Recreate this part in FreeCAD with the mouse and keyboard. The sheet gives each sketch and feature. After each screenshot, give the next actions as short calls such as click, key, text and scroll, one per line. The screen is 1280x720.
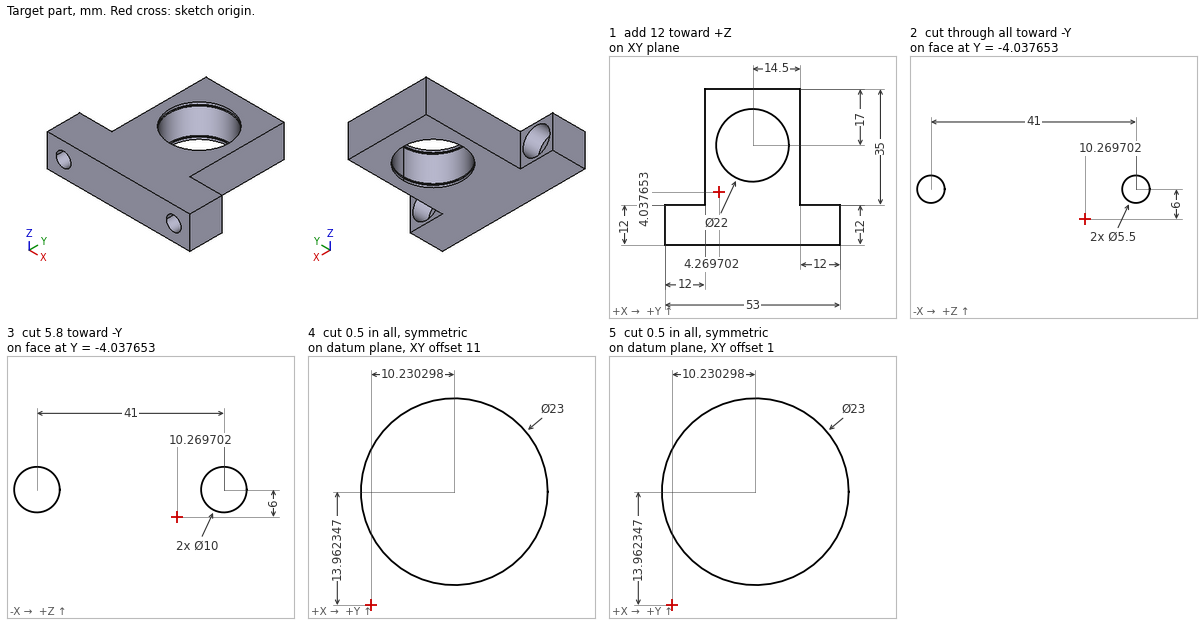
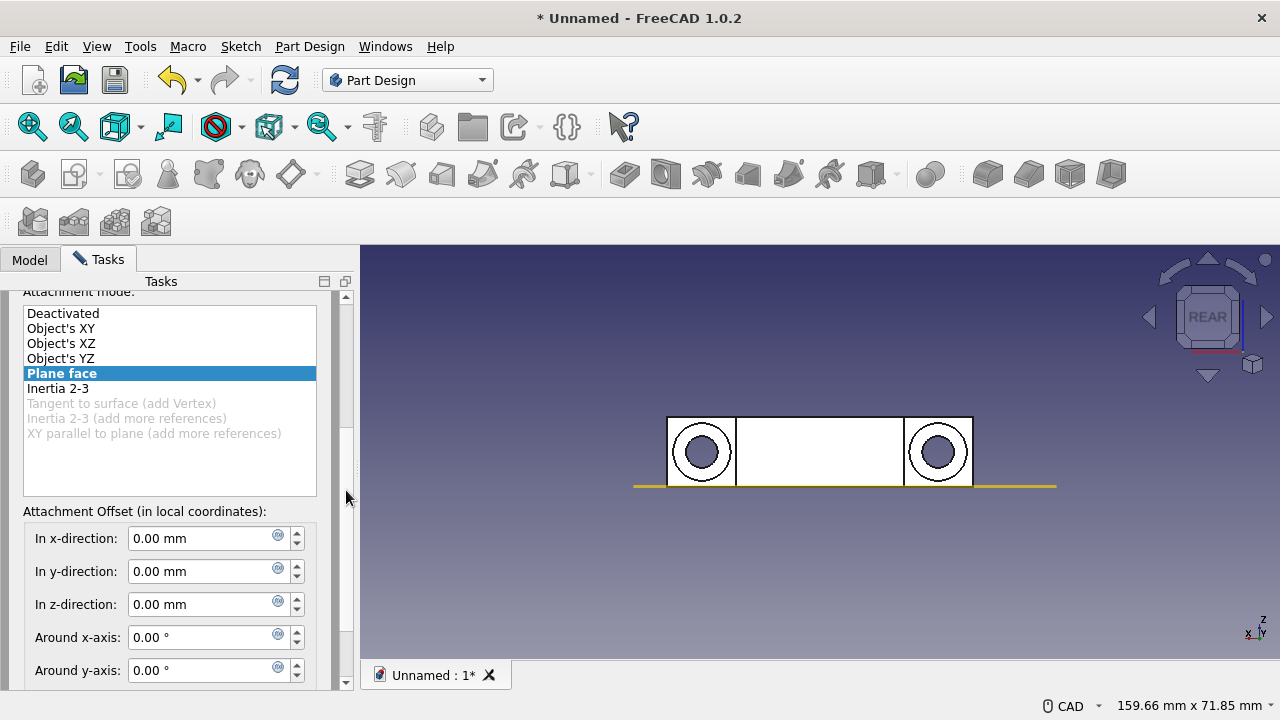
triple_click(210, 604)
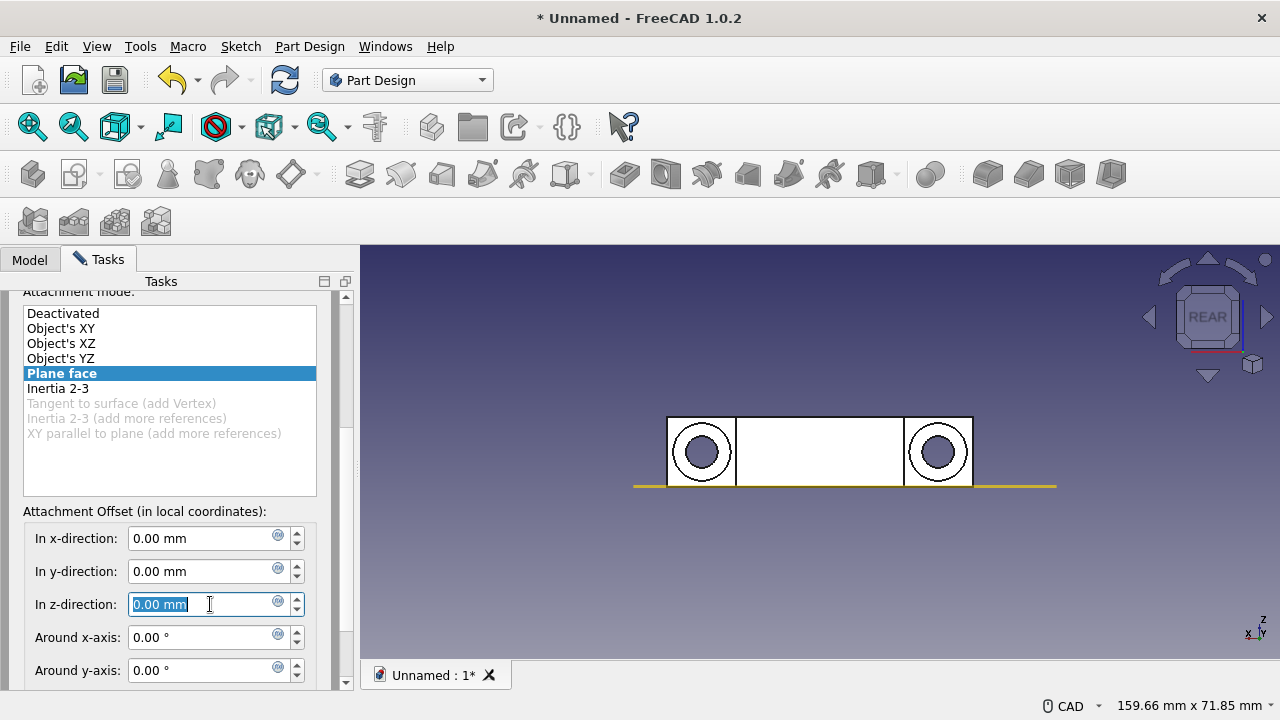
text(1)
key(Tab)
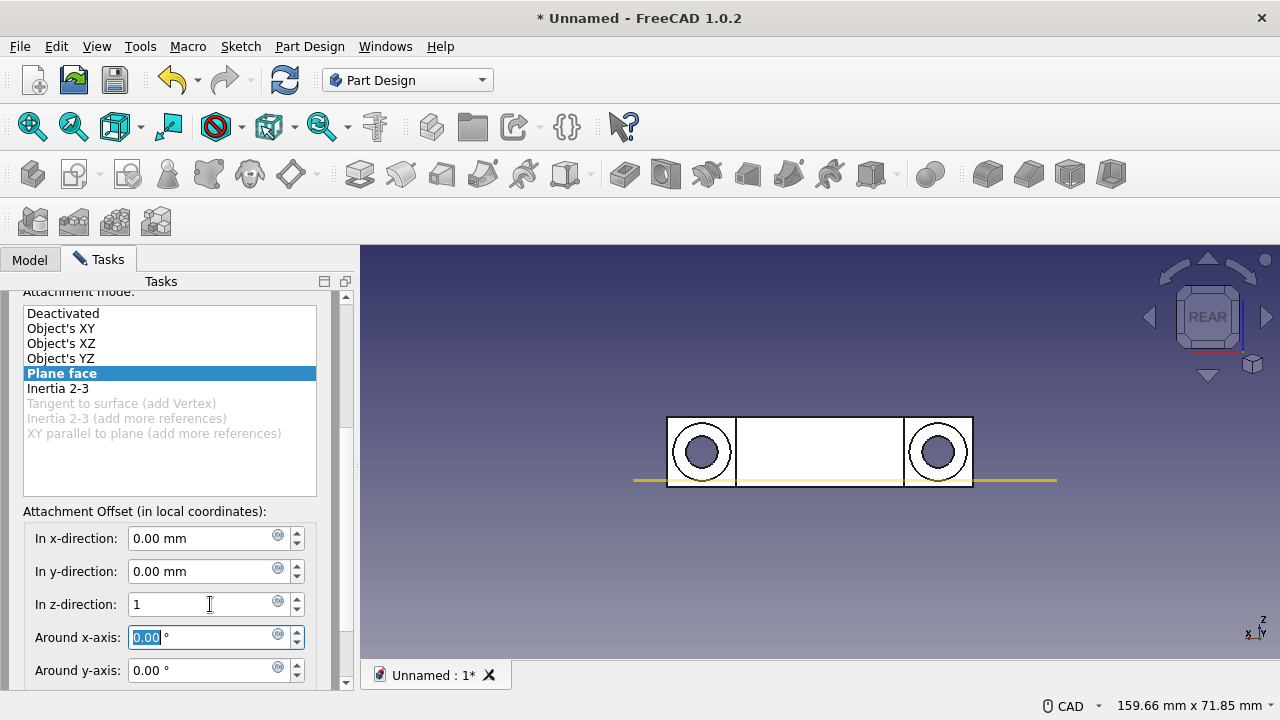
scroll(346, 490, up, 5)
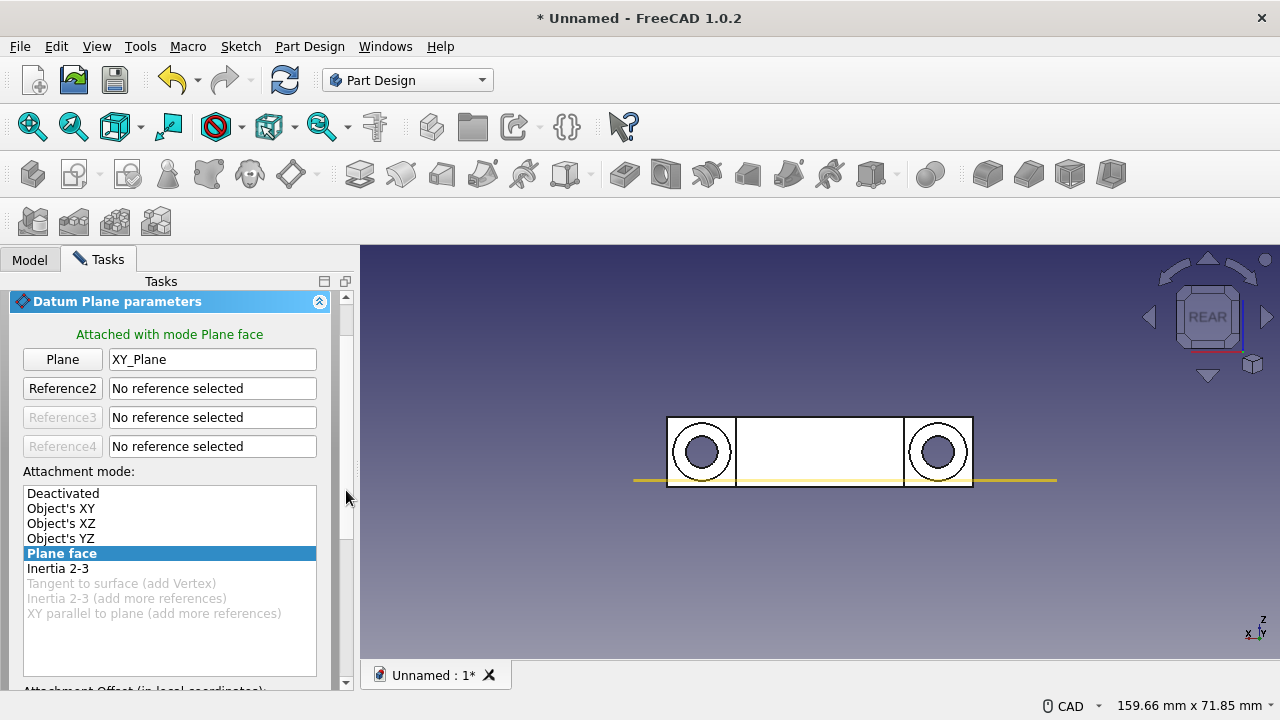
click(127, 320)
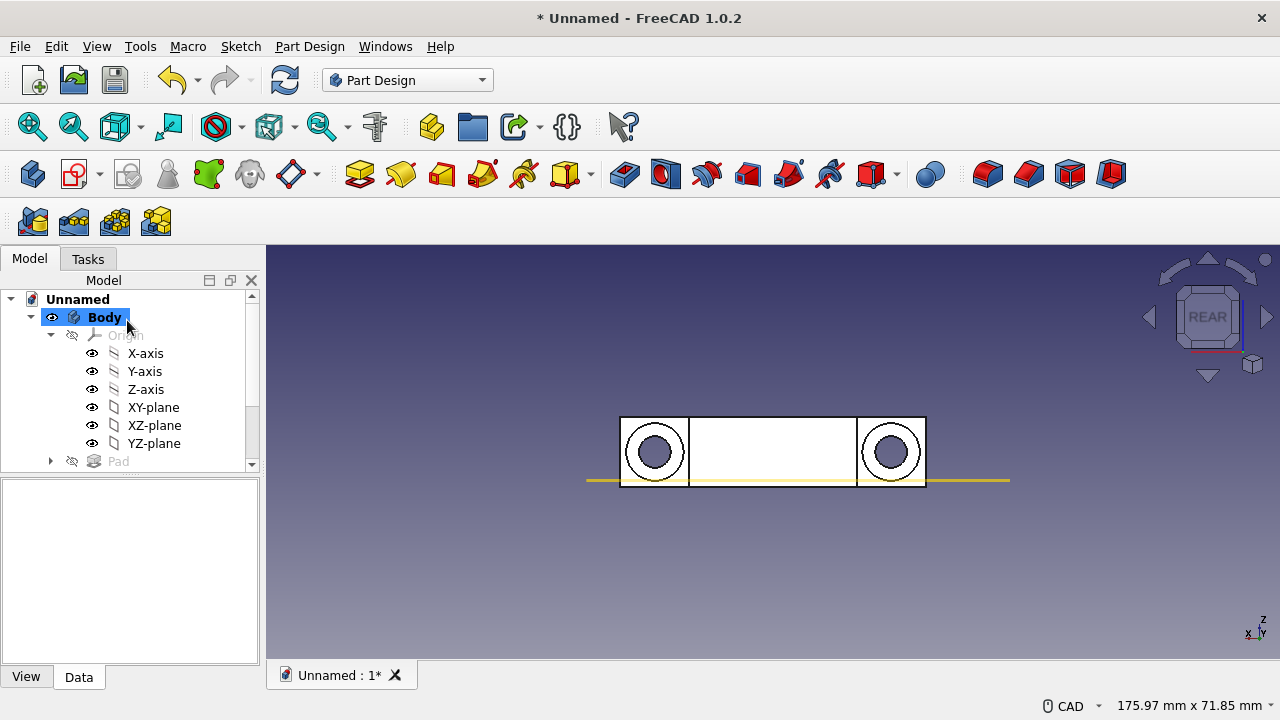
scroll(101, 385, down, 3)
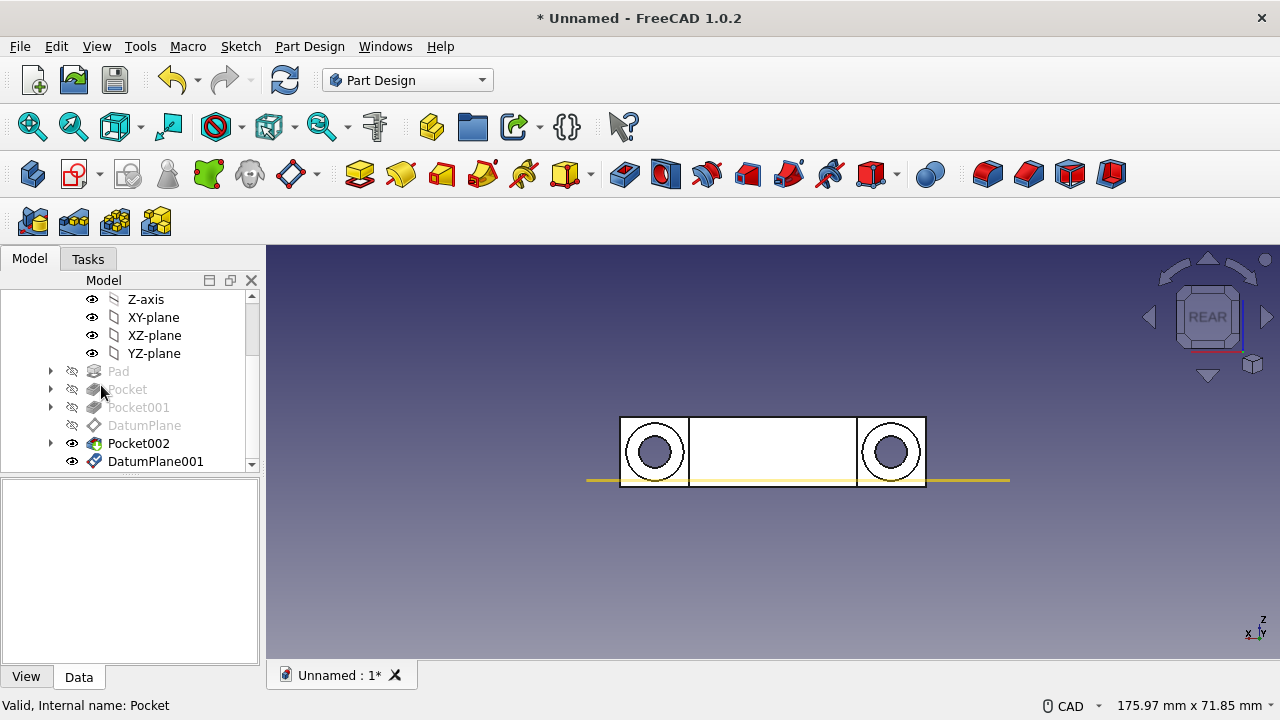
click(117, 461)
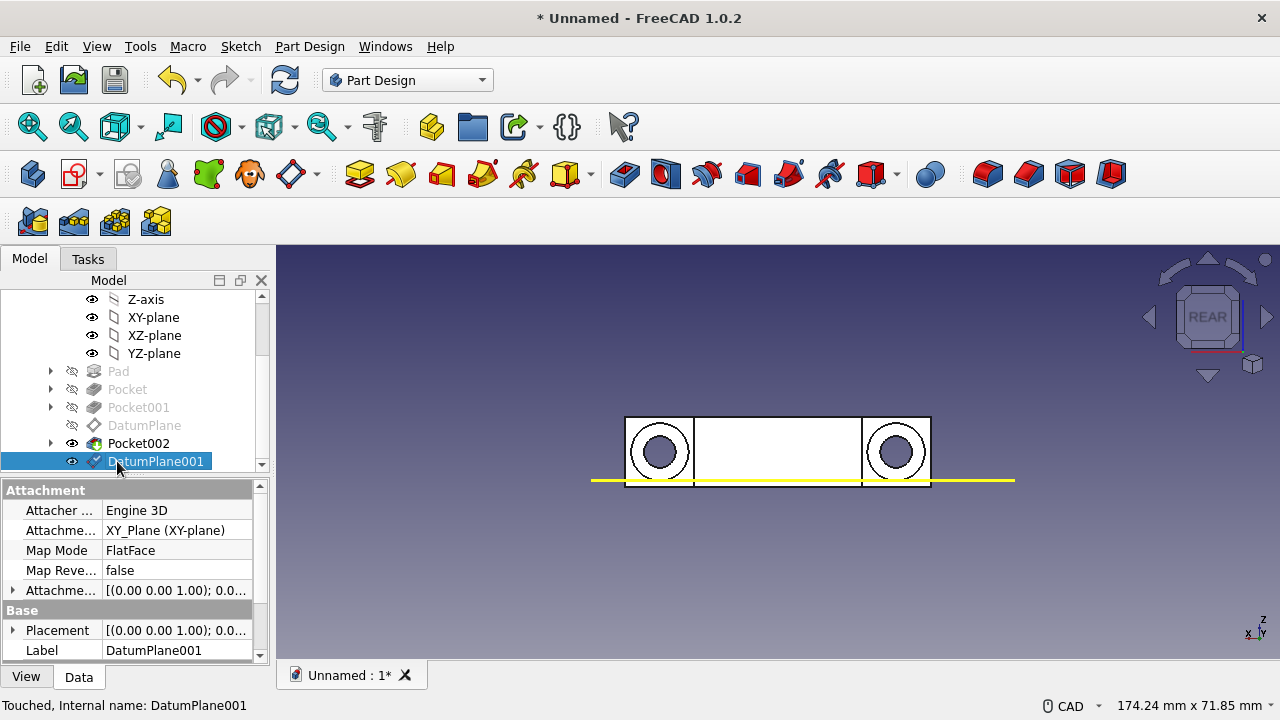
click(74, 174)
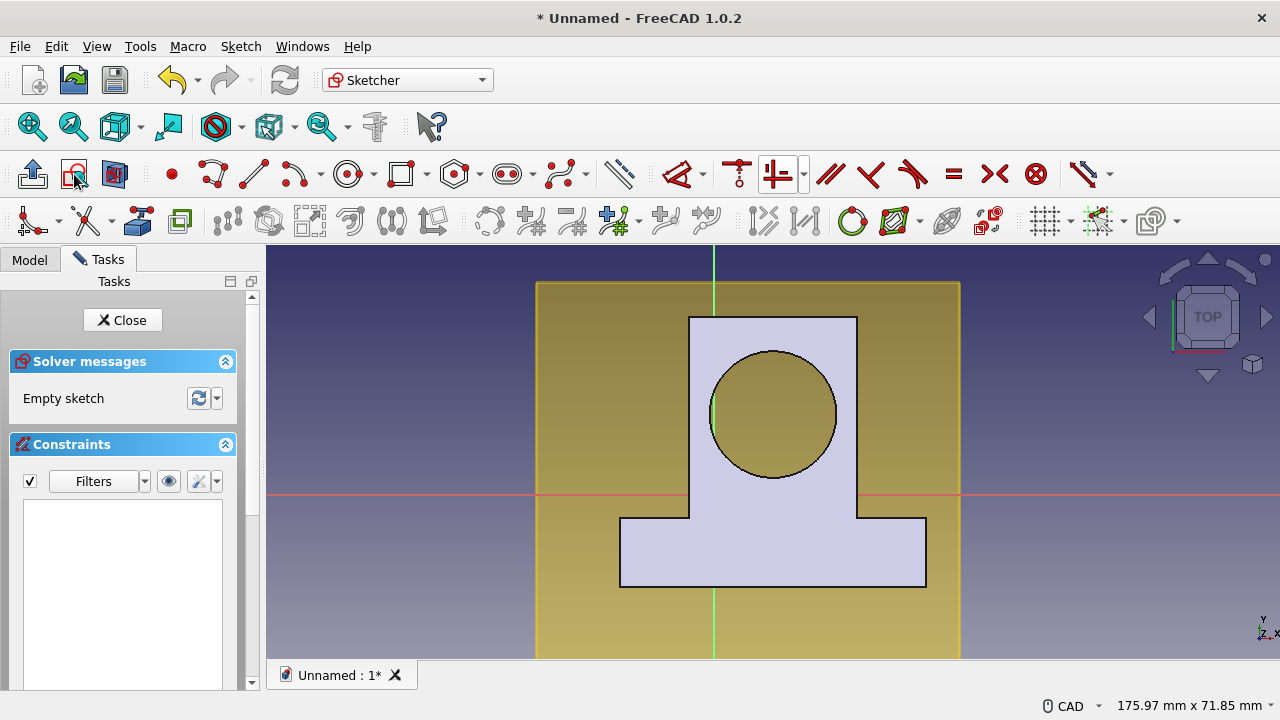
click(115, 174)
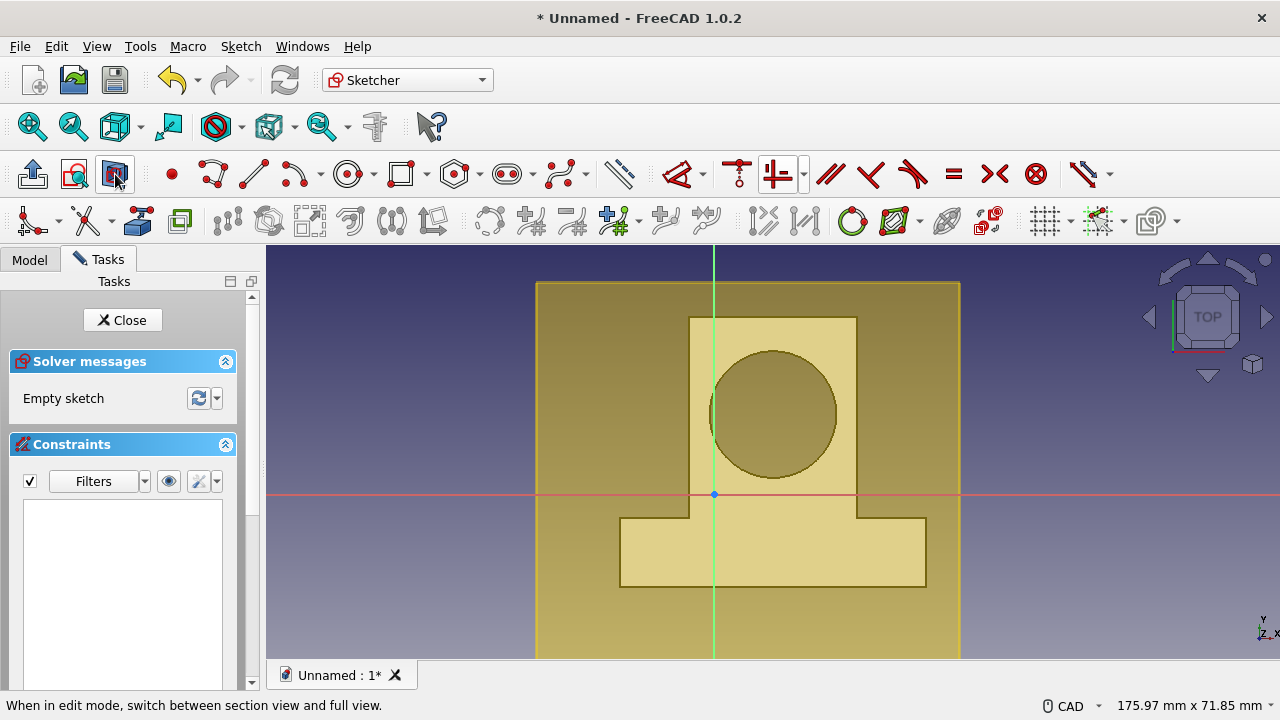
scroll(856, 385, up, 3)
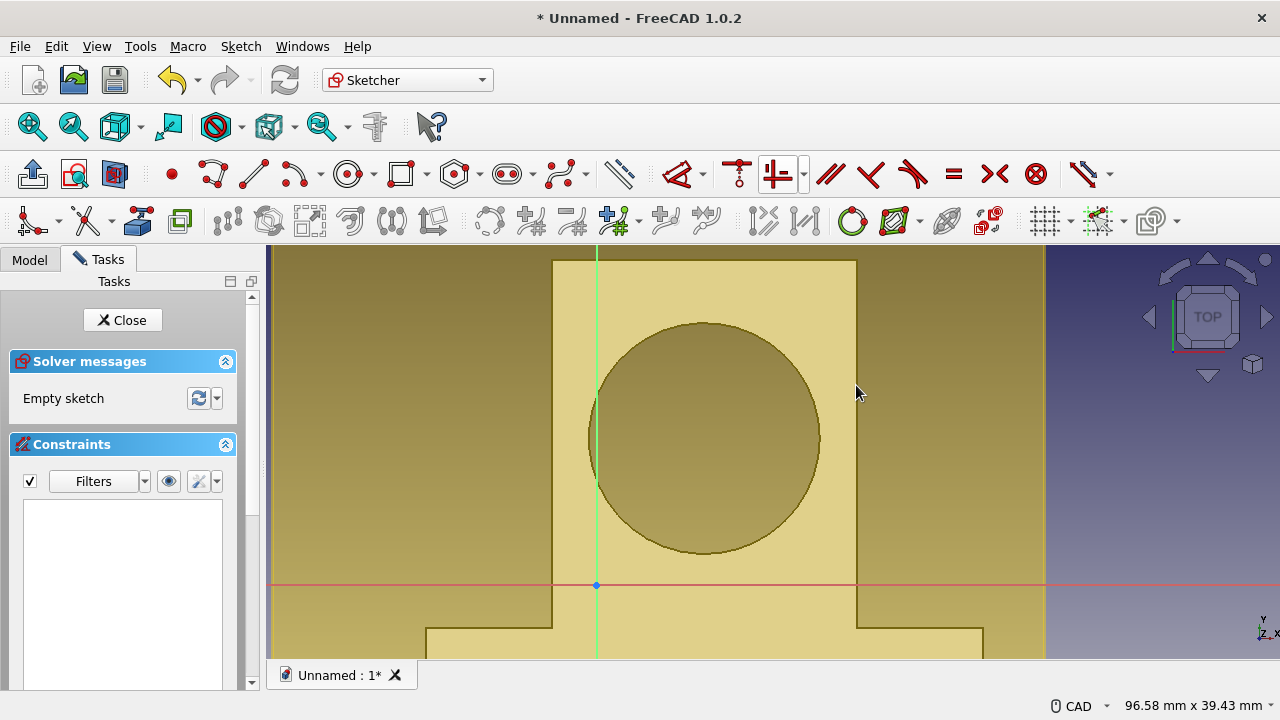
click(348, 174)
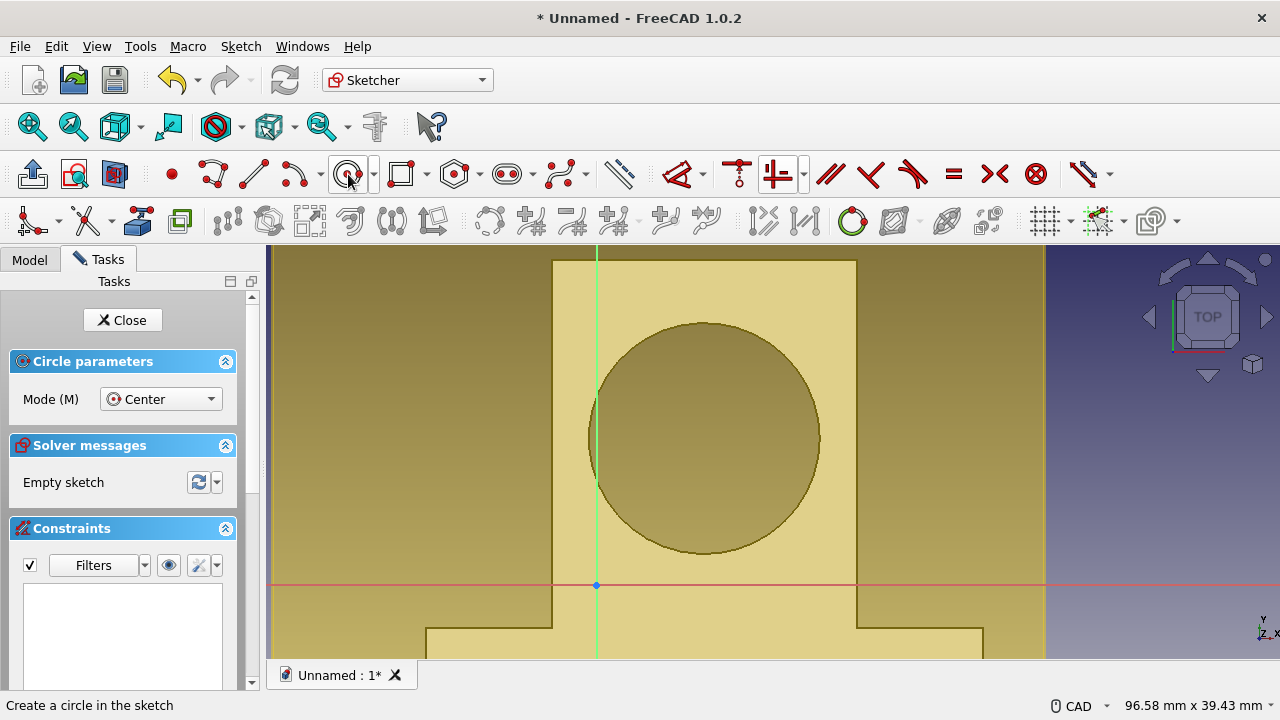
click(704, 439)
click(790, 353)
key(Escape)